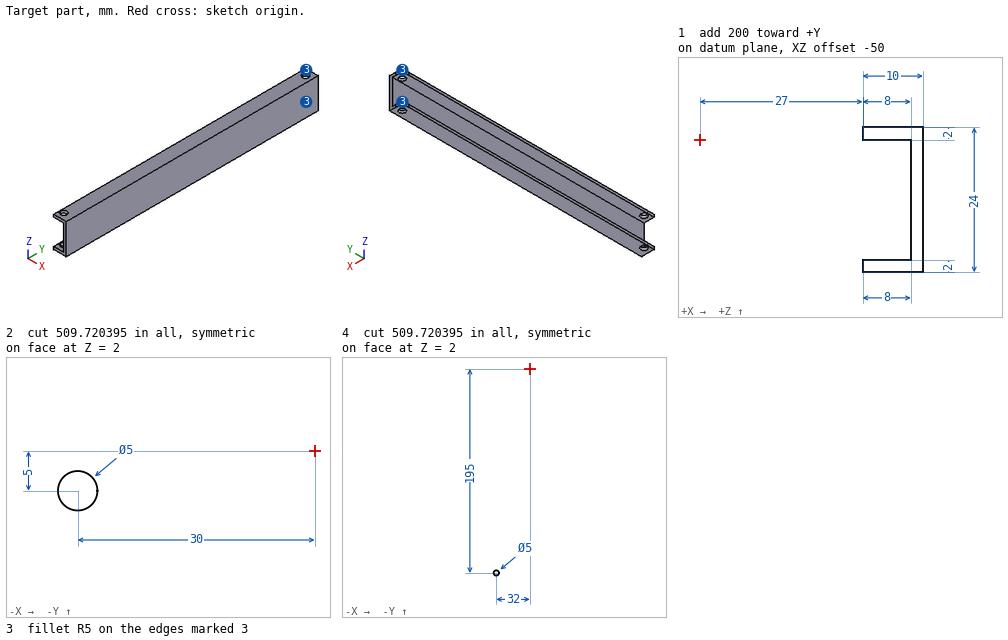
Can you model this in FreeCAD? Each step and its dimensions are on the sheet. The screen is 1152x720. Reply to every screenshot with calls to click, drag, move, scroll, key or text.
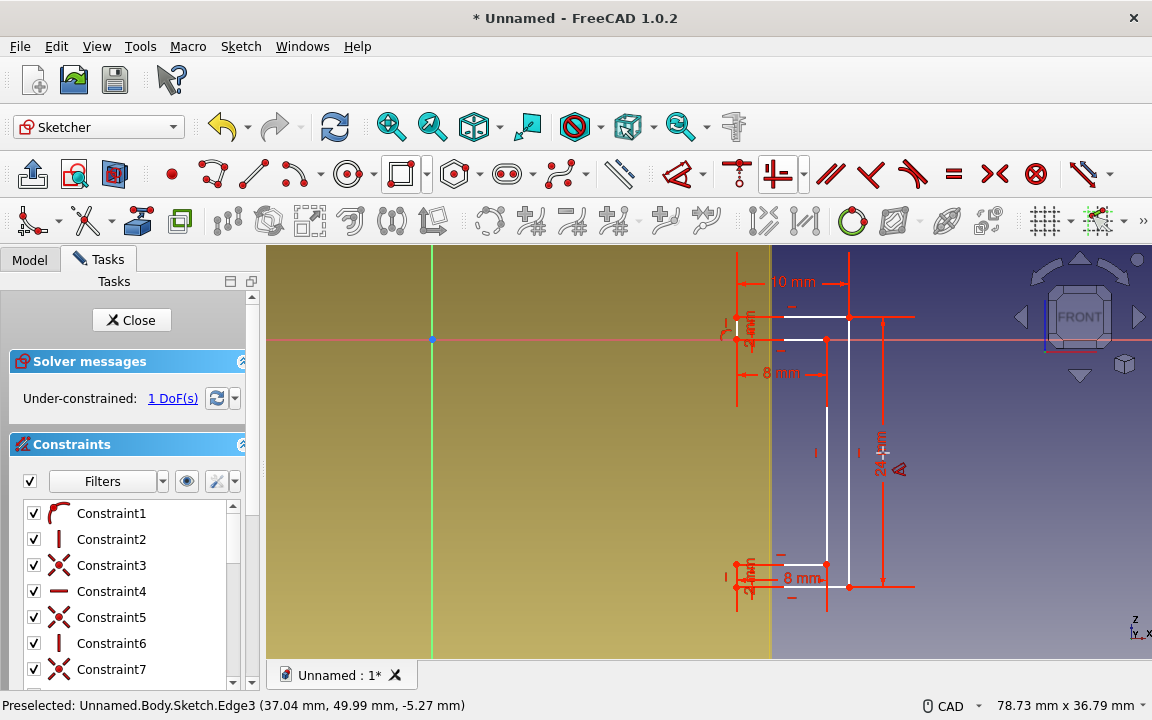
click(737, 340)
click(585, 306)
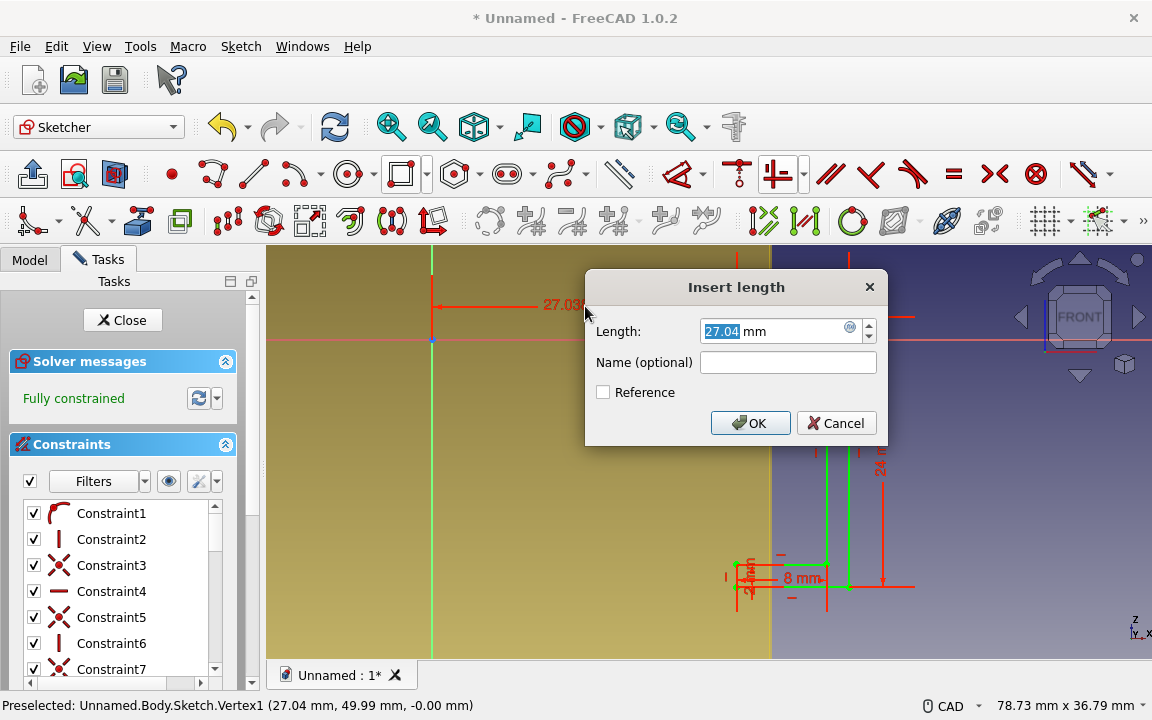
text(27)
key(Return)
key(Escape)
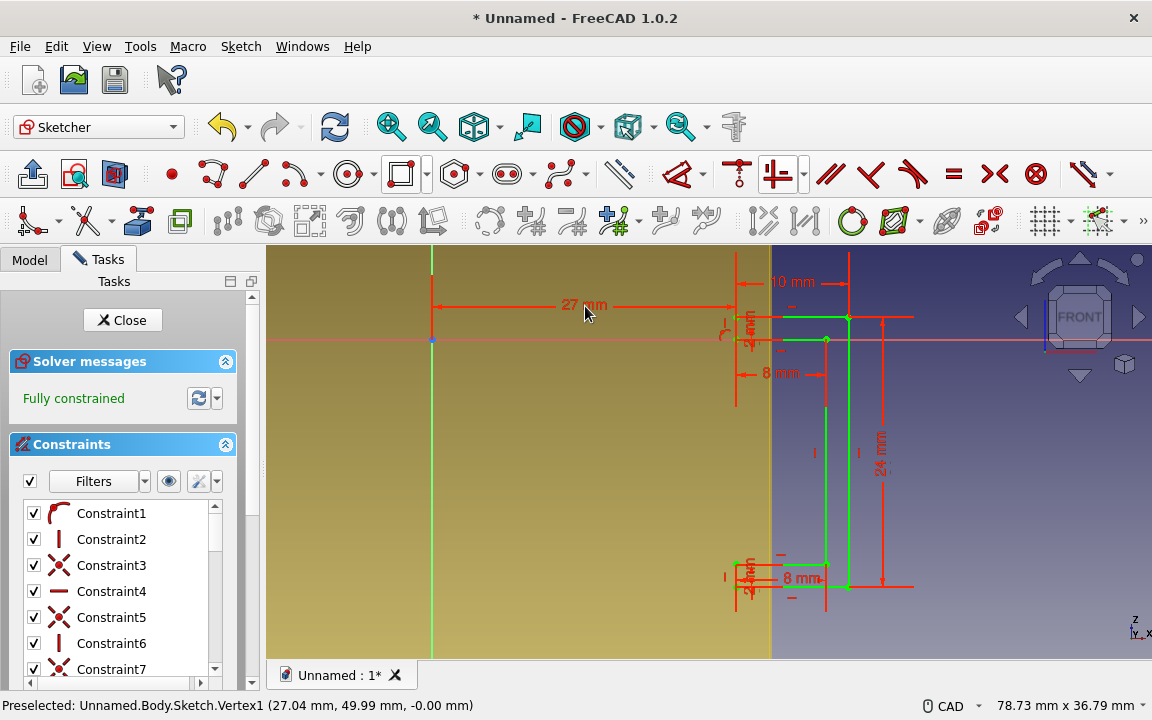
click(123, 320)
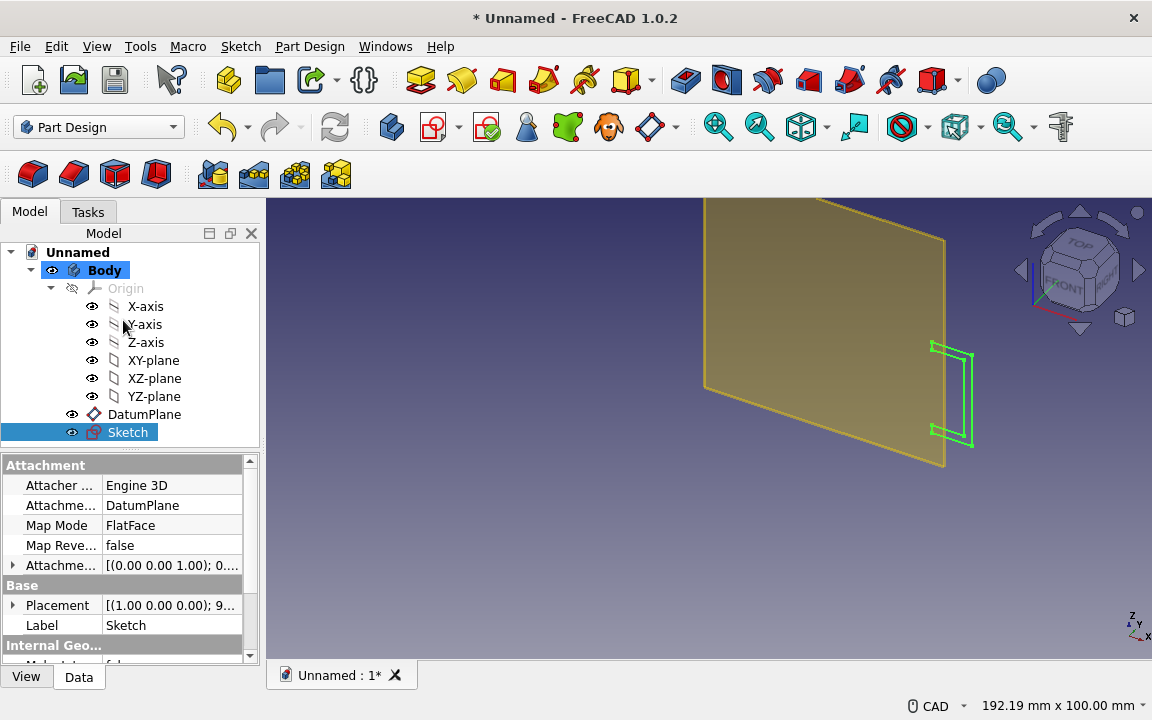
click(421, 80)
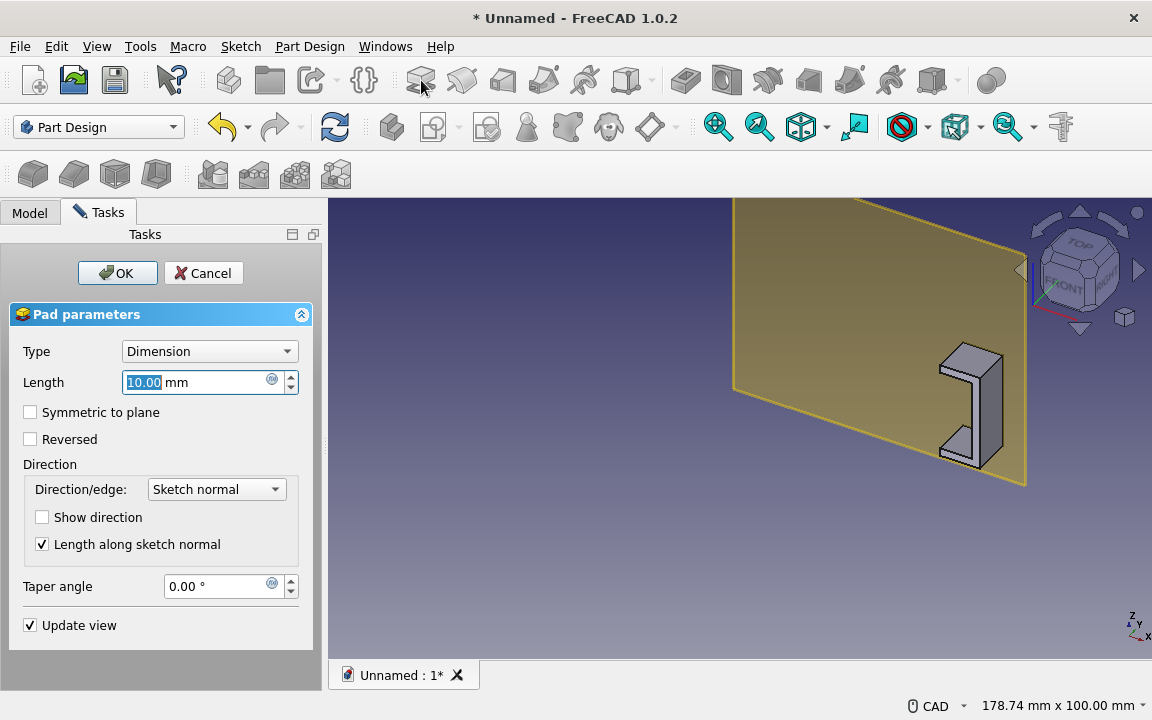
text(200)
key(Tab)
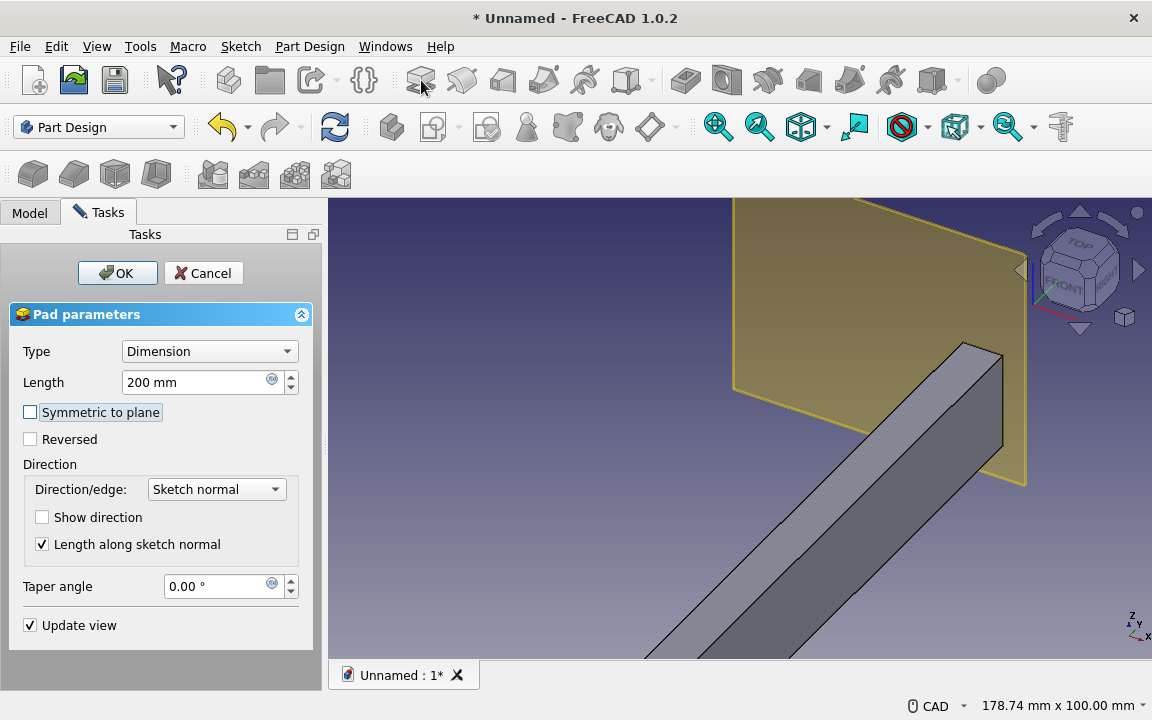
click(31, 439)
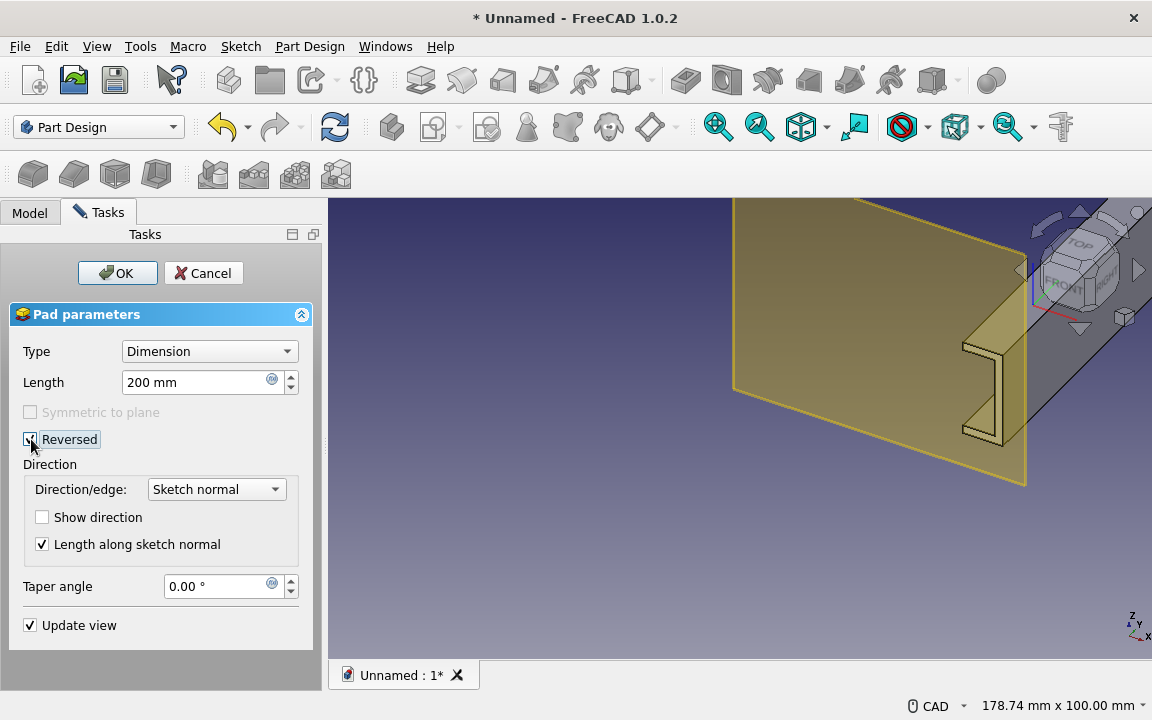
click(118, 273)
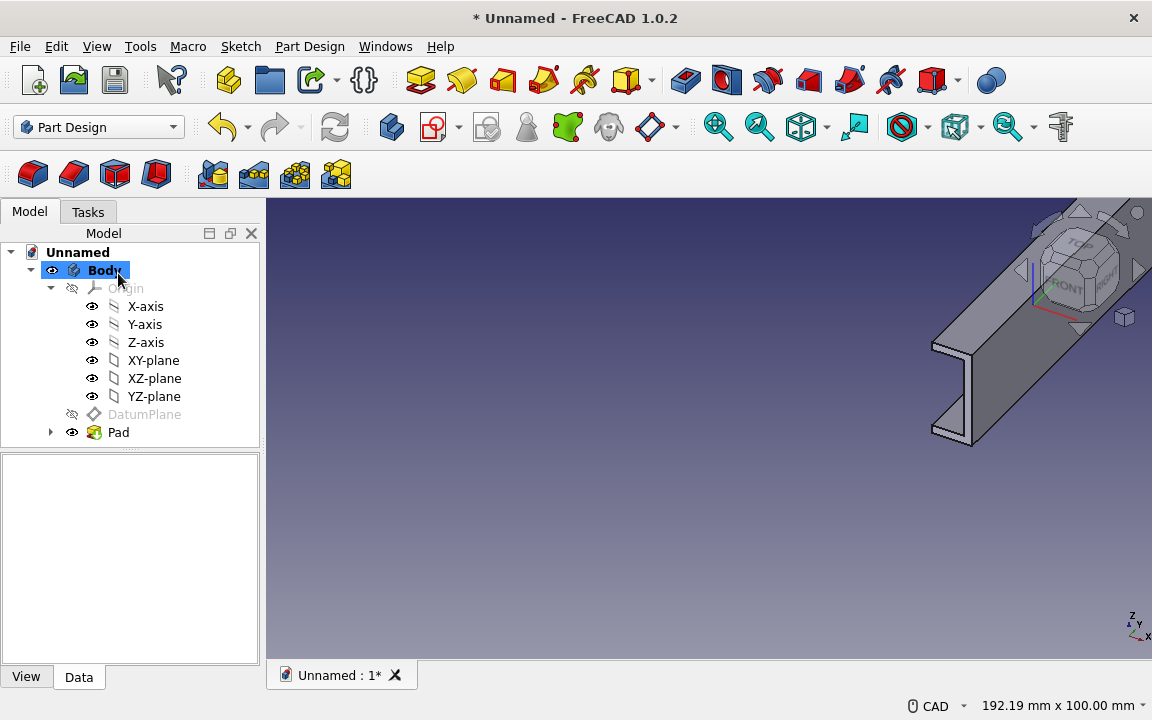
click(719, 128)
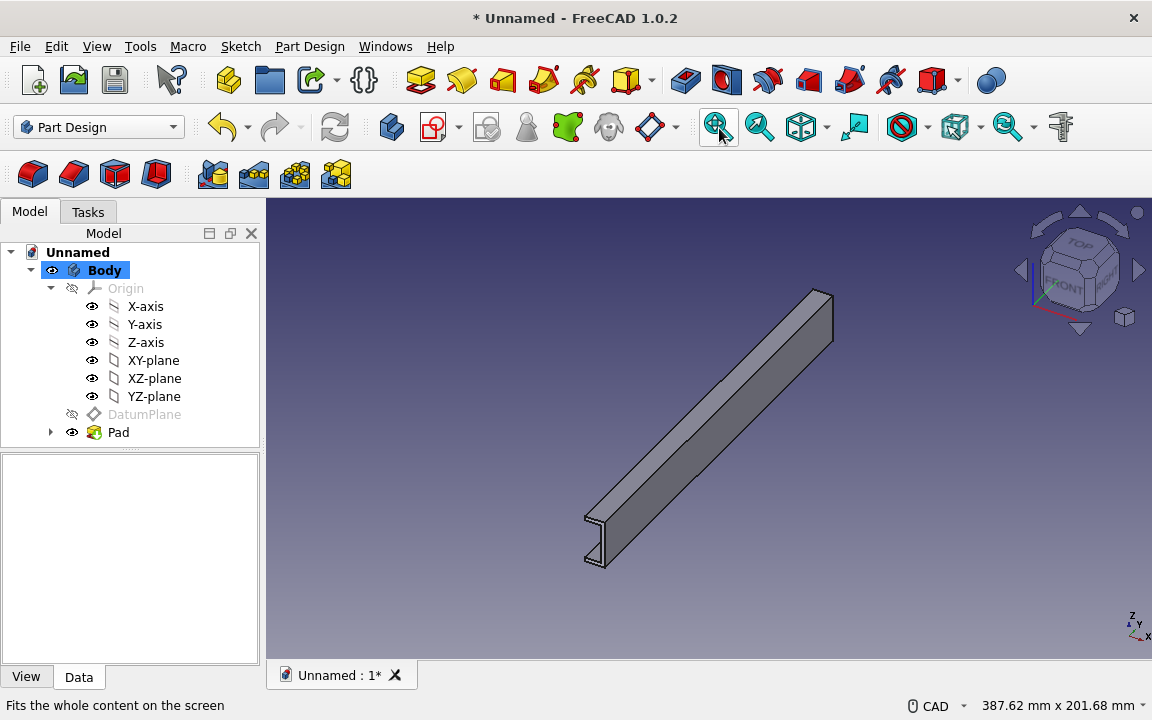
click(774, 340)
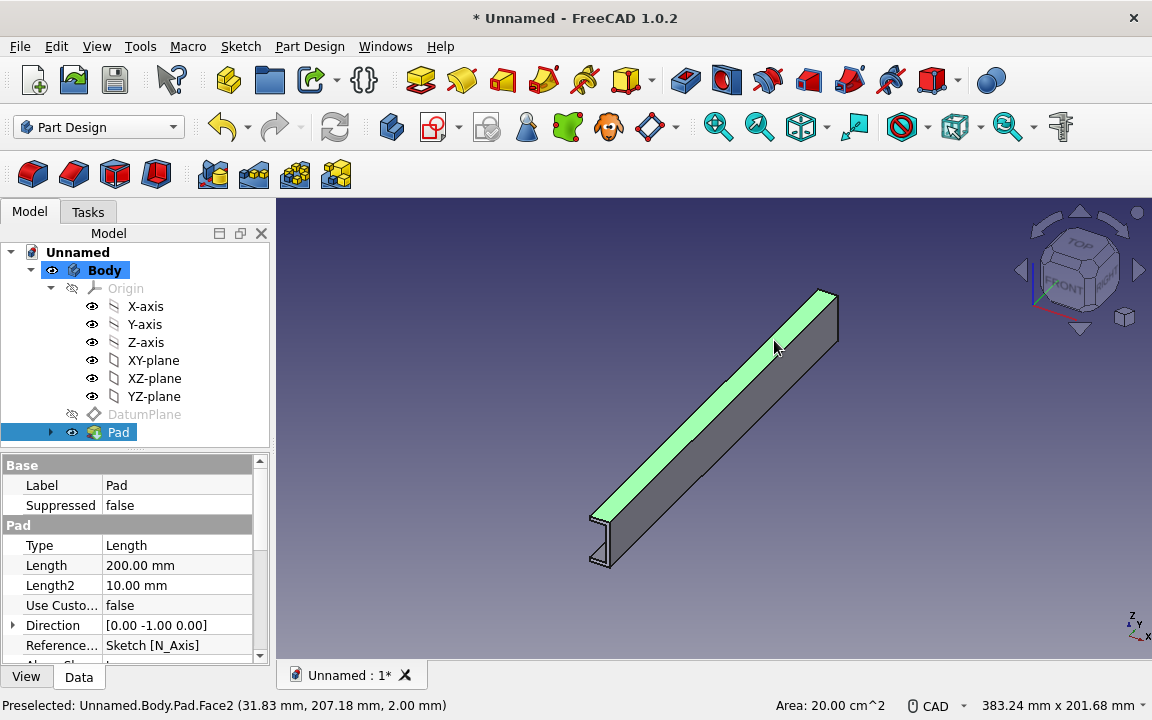
click(432, 128)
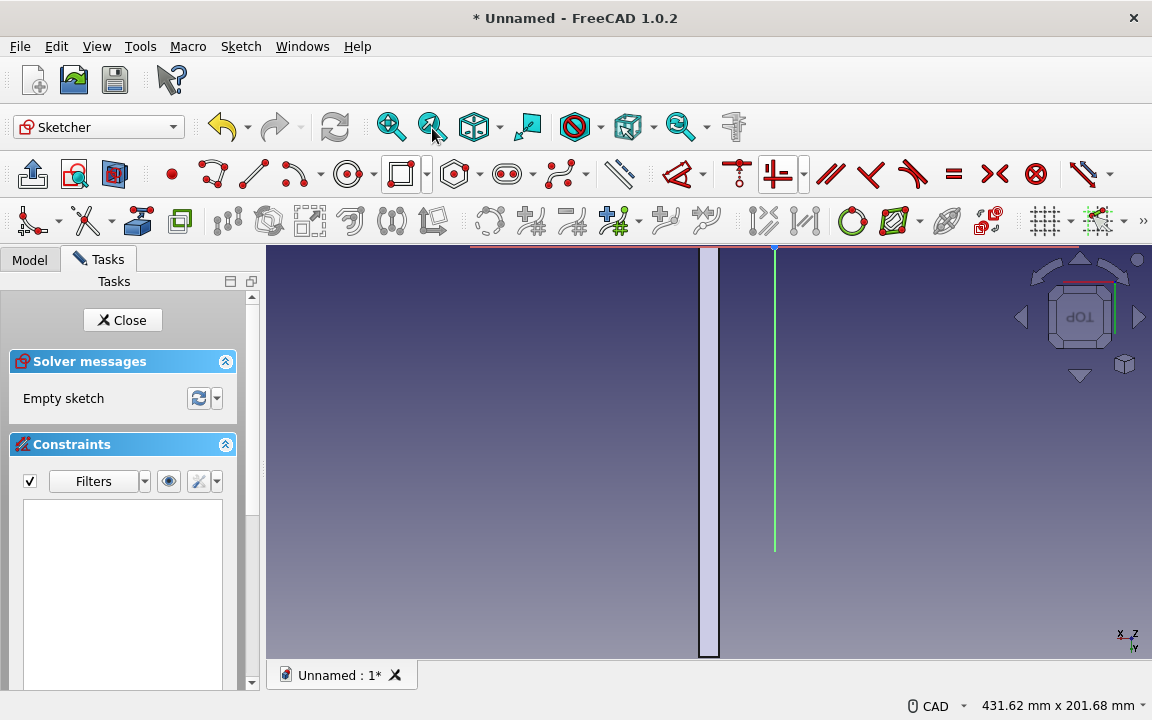
scroll(640, 452, down, 5)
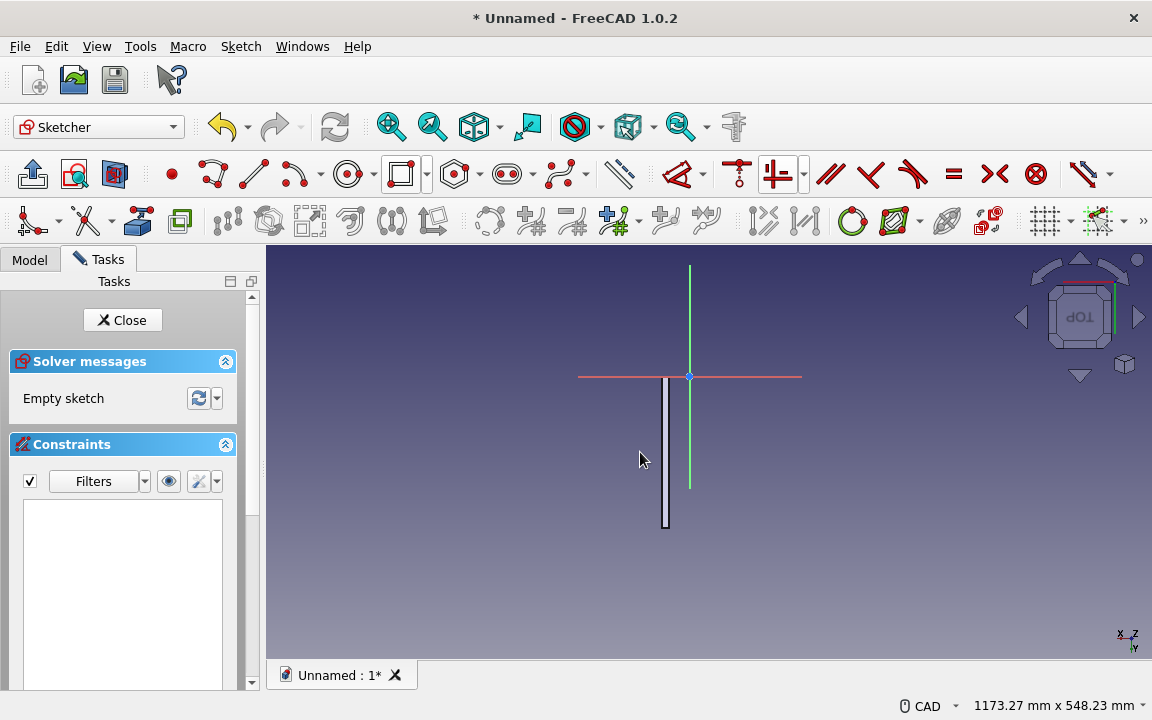
scroll(669, 377, up, 15)